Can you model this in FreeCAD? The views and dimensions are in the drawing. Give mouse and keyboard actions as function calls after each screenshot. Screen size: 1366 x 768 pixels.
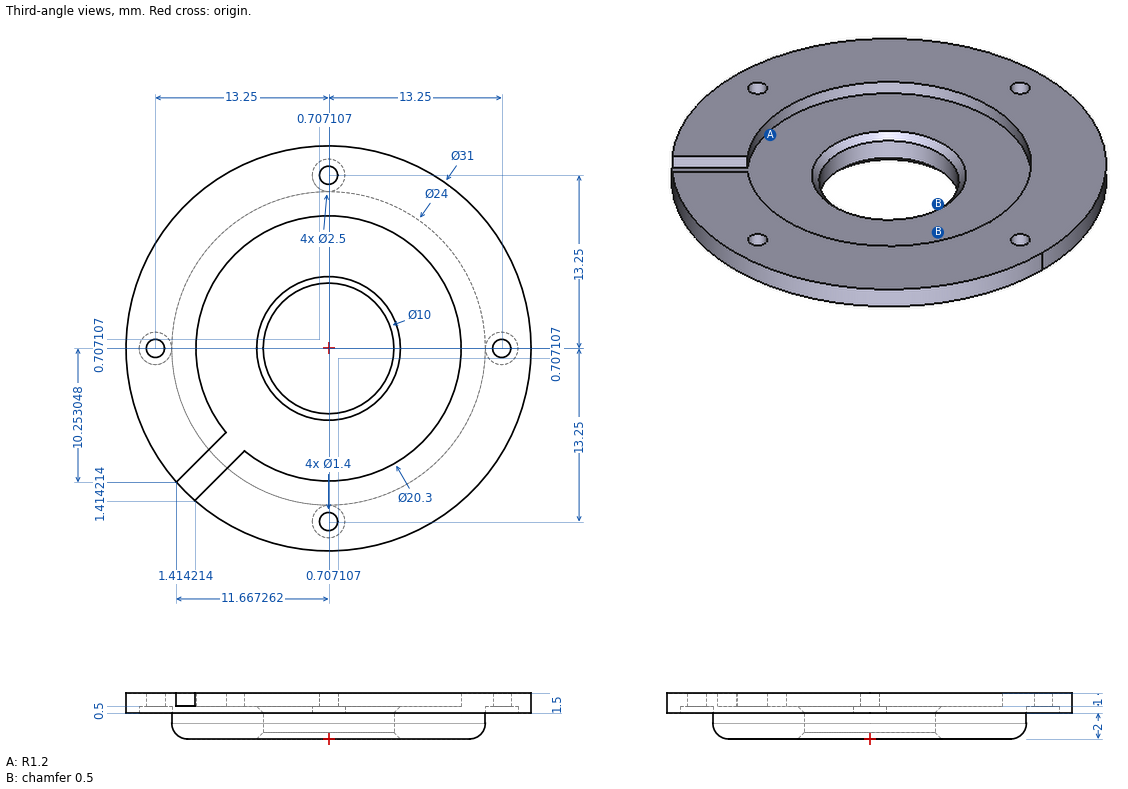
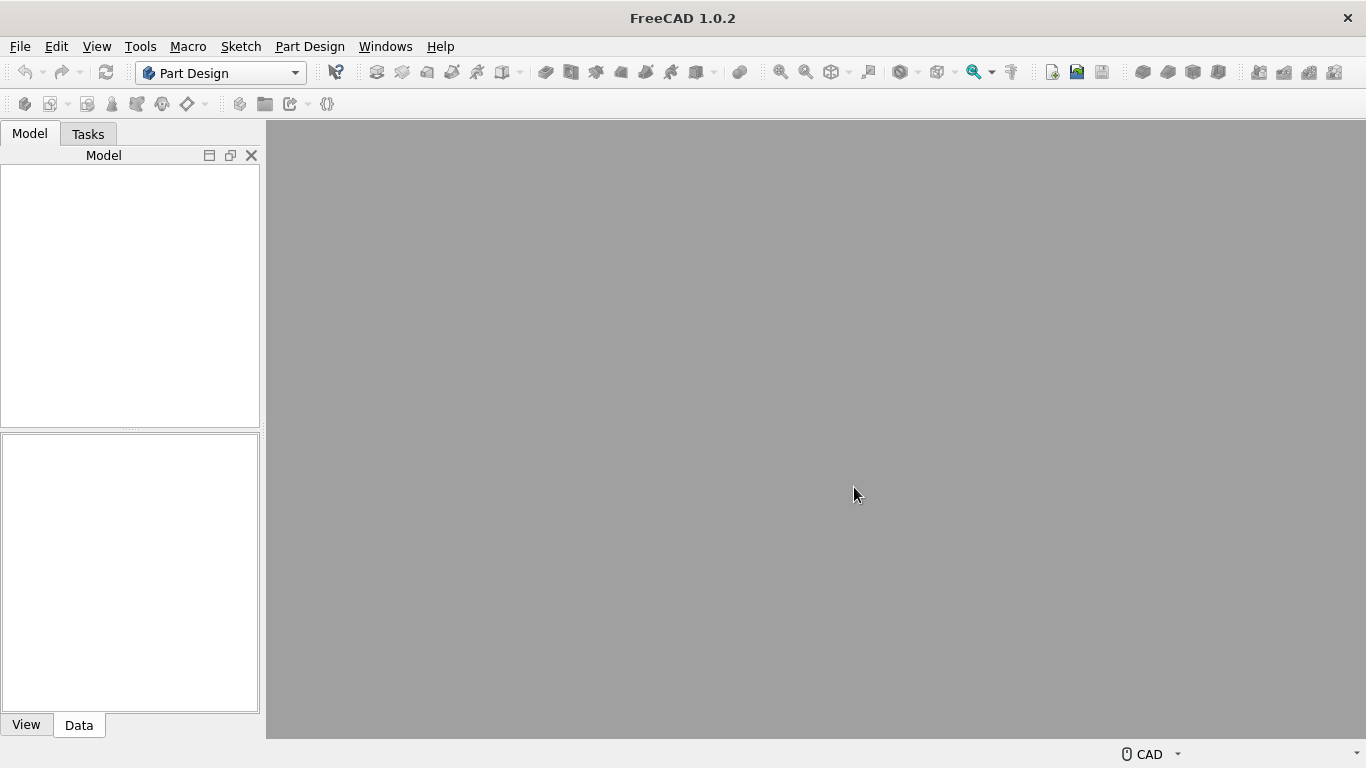
click(1052, 72)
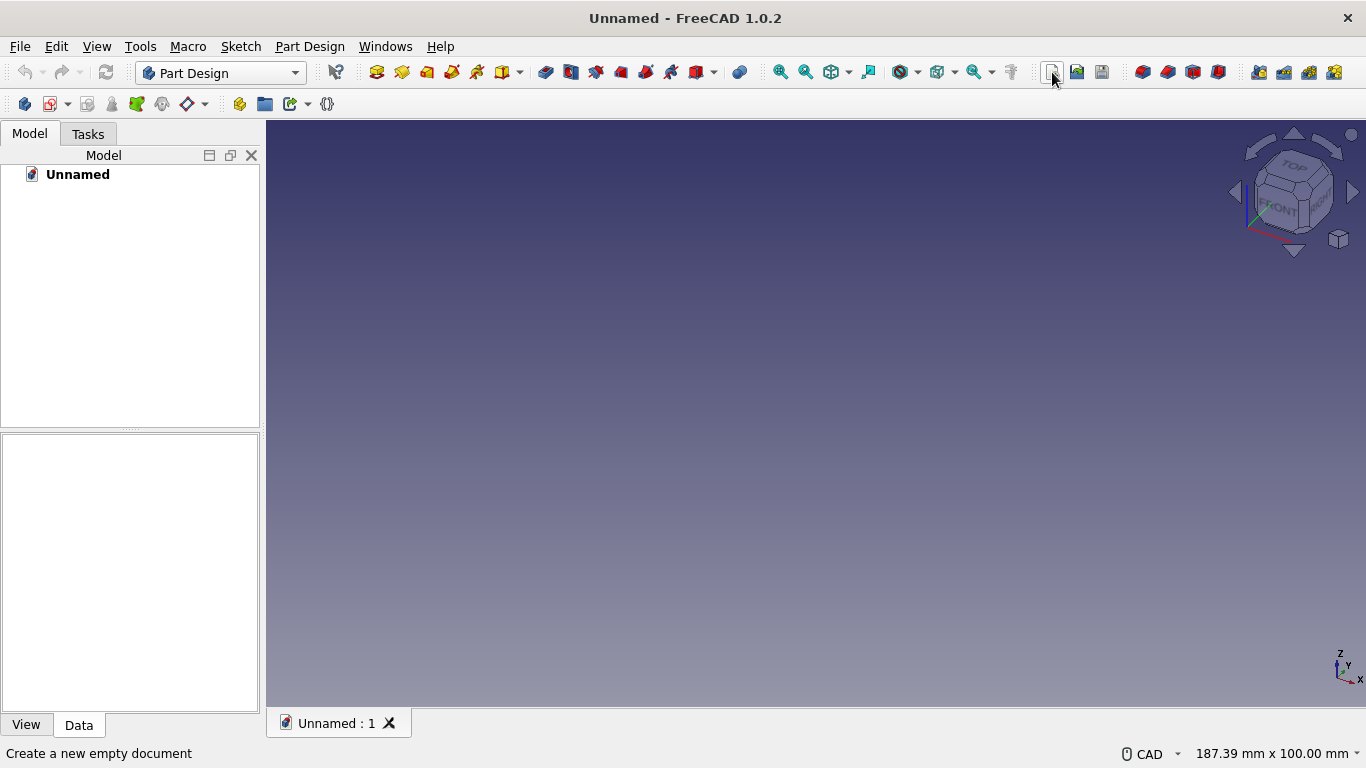
click(50, 104)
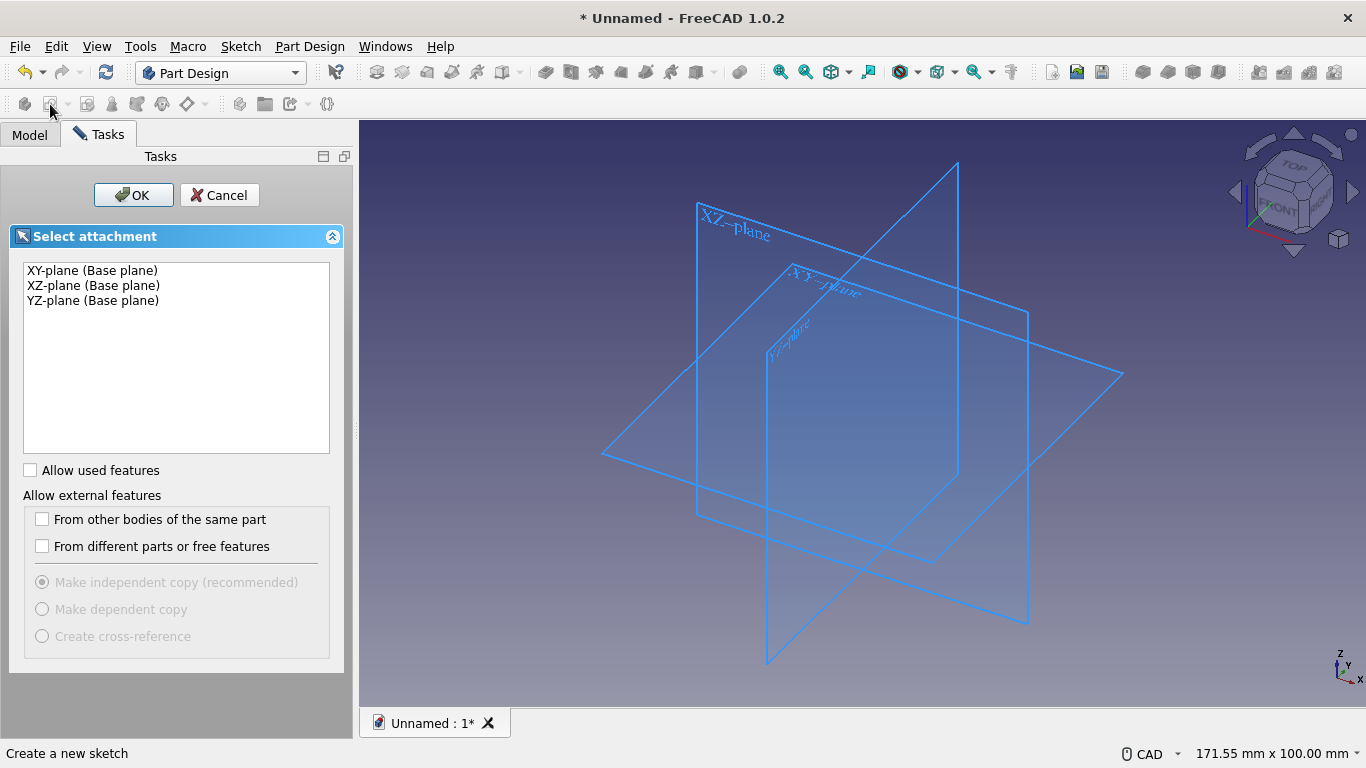
click(84, 270)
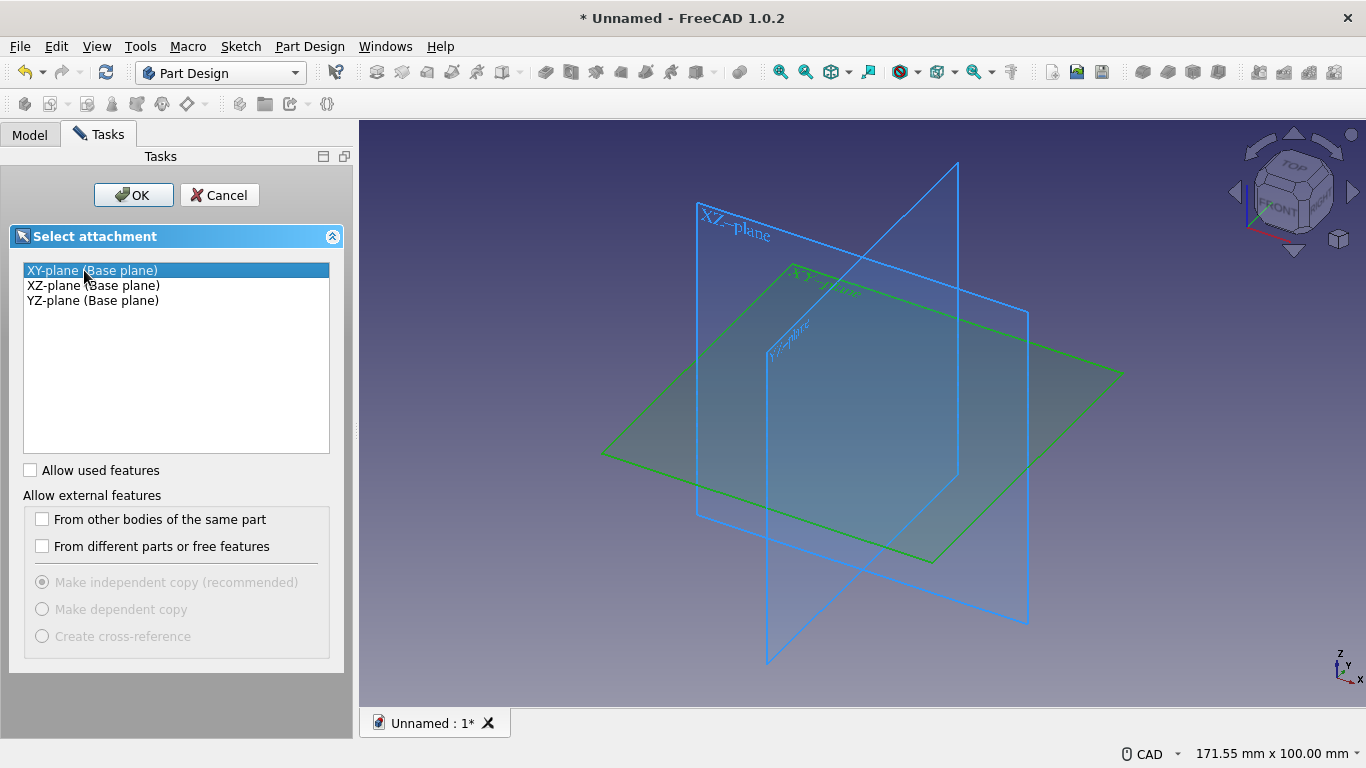
click(134, 195)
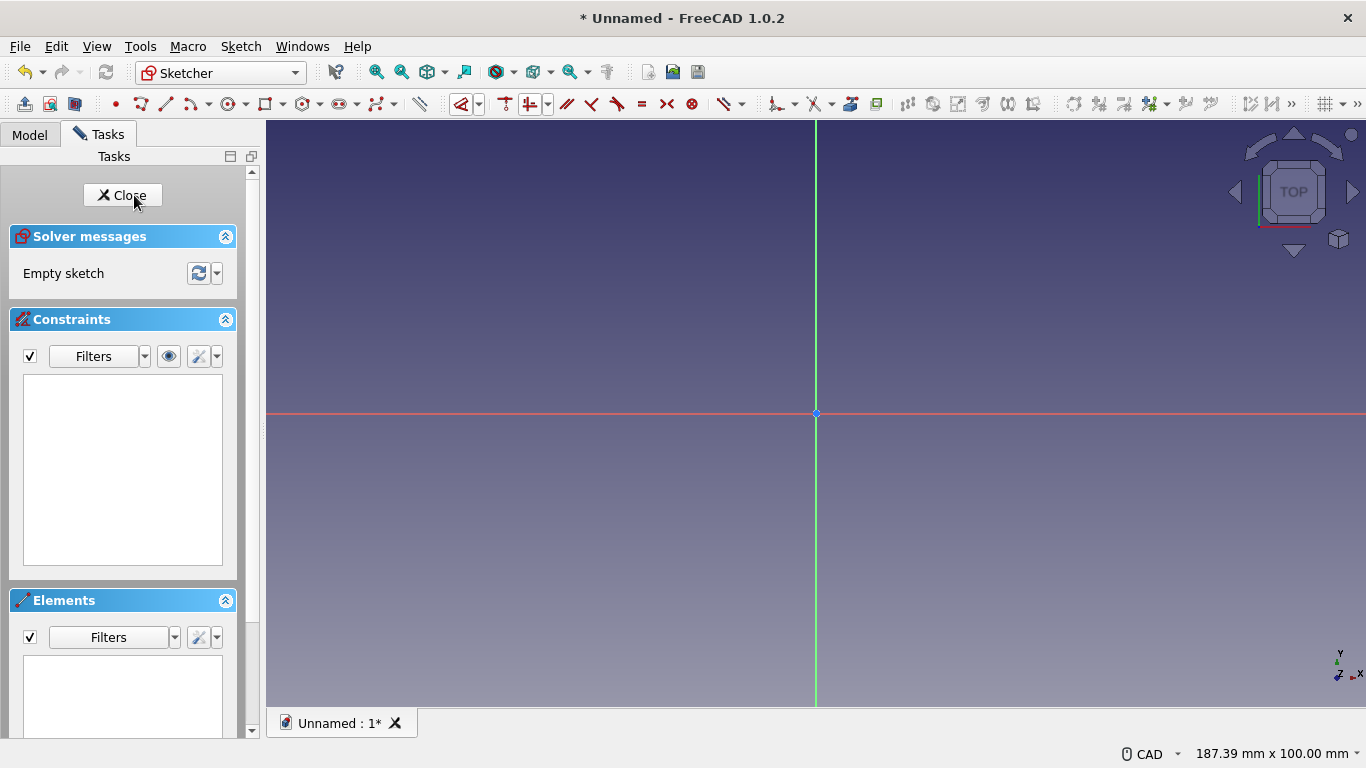
scroll(856, 414, up, 5)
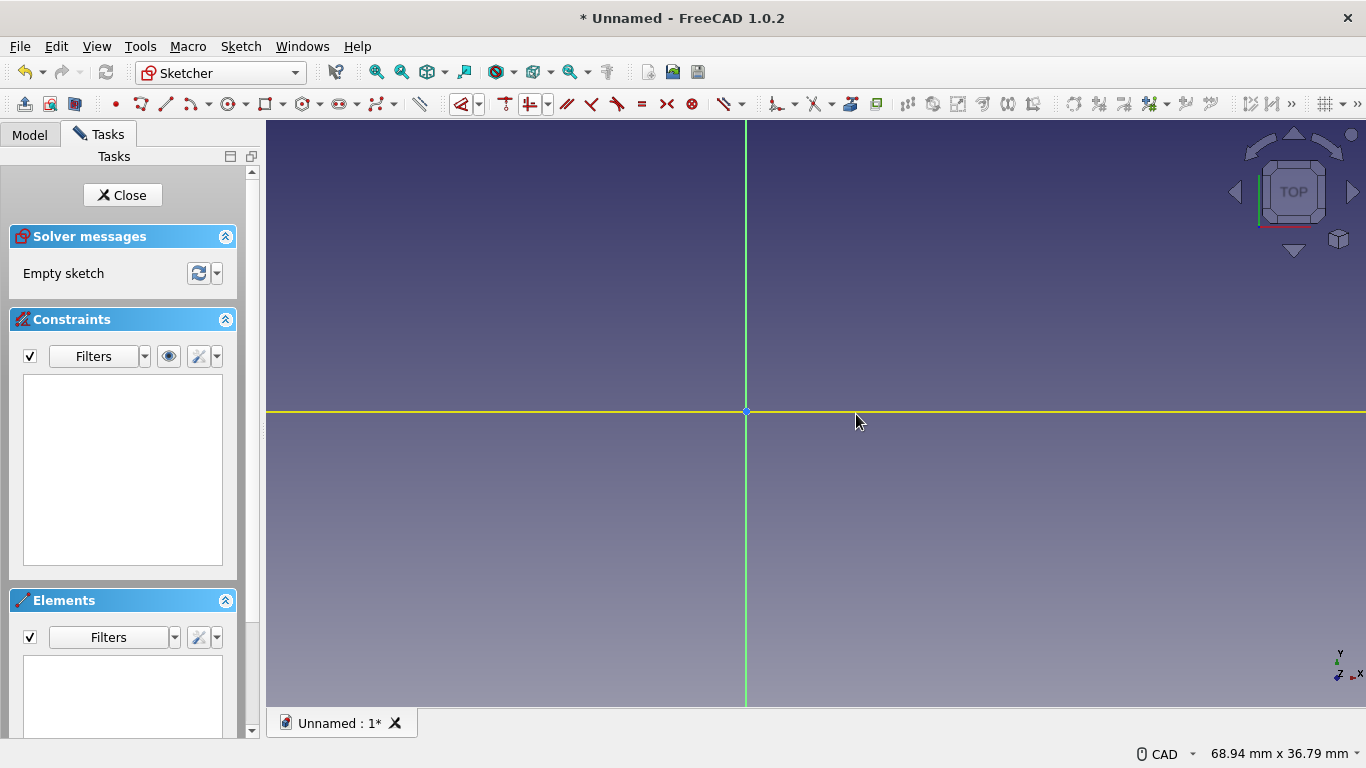
key(g)
key(c)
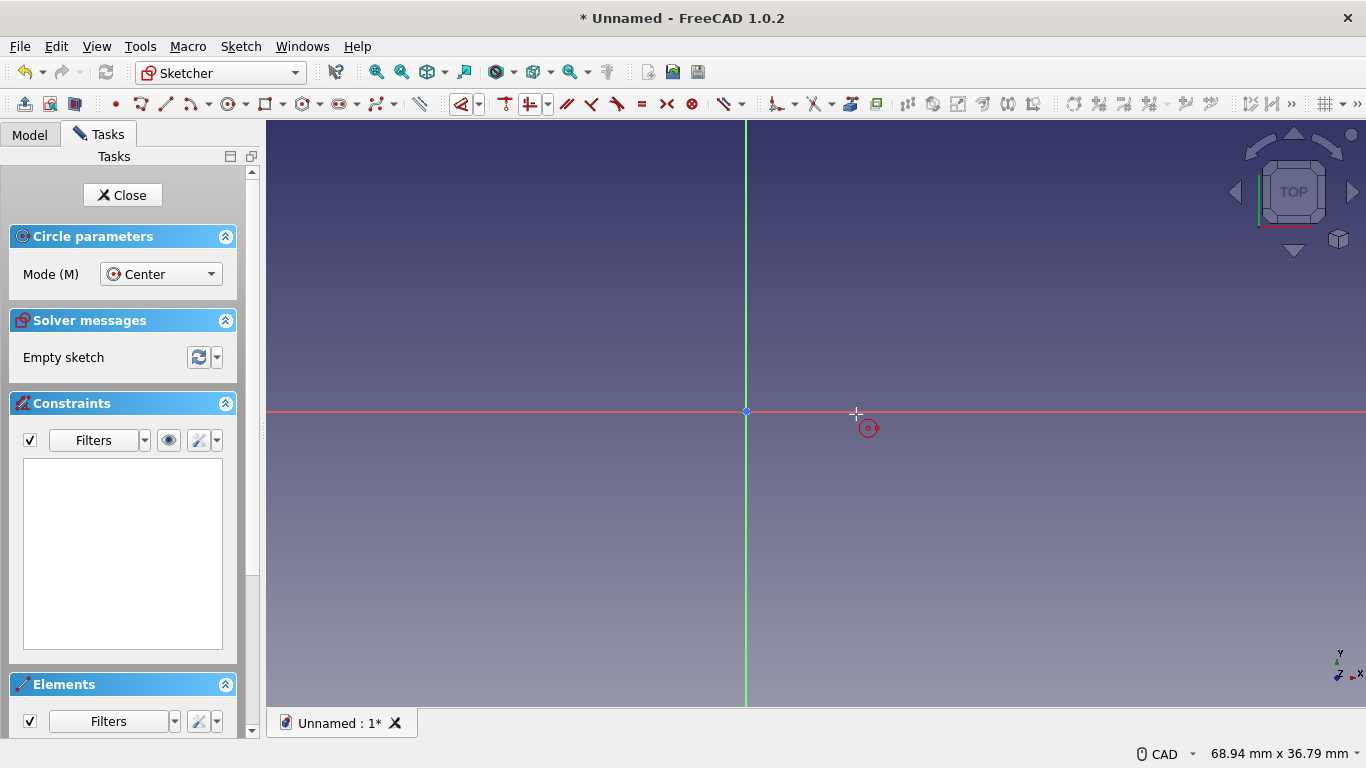
click(746, 412)
move(882, 276)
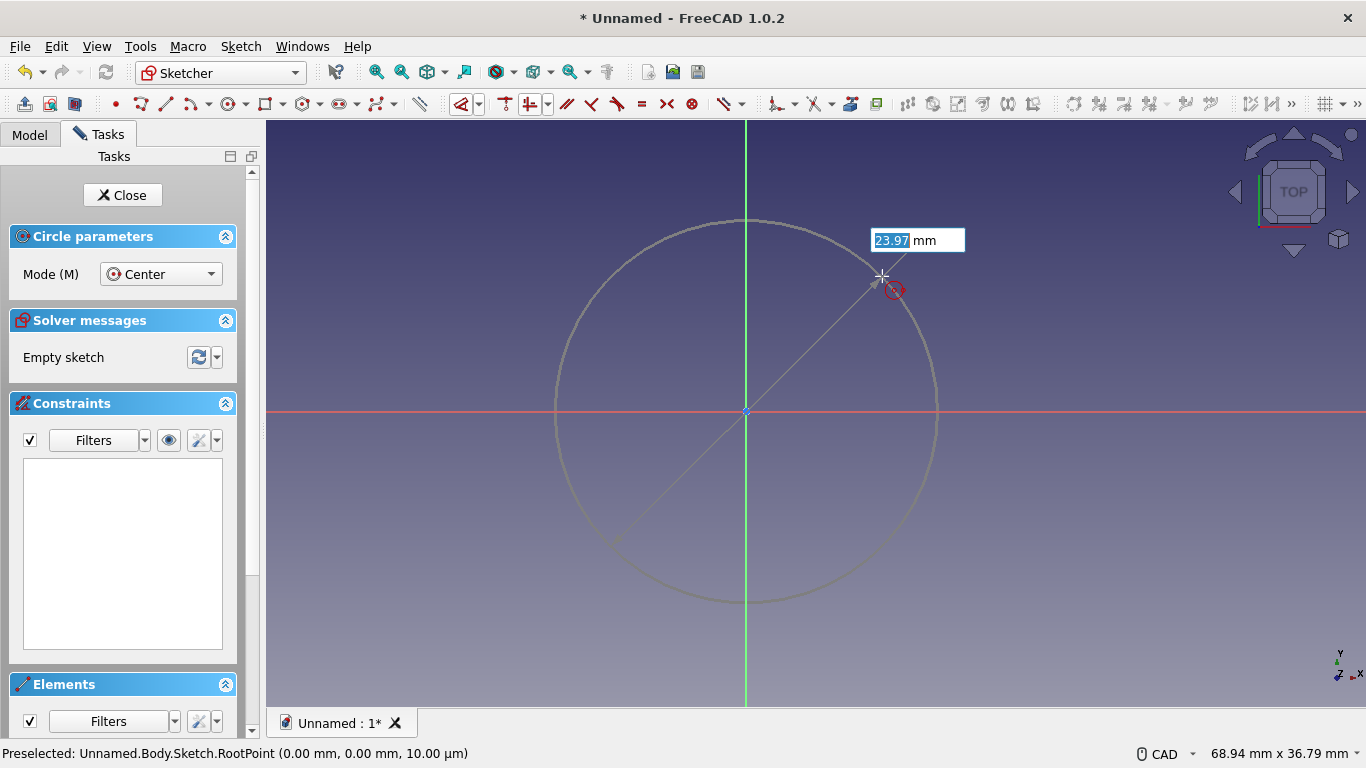
text(24)
key(Return)
key(Escape)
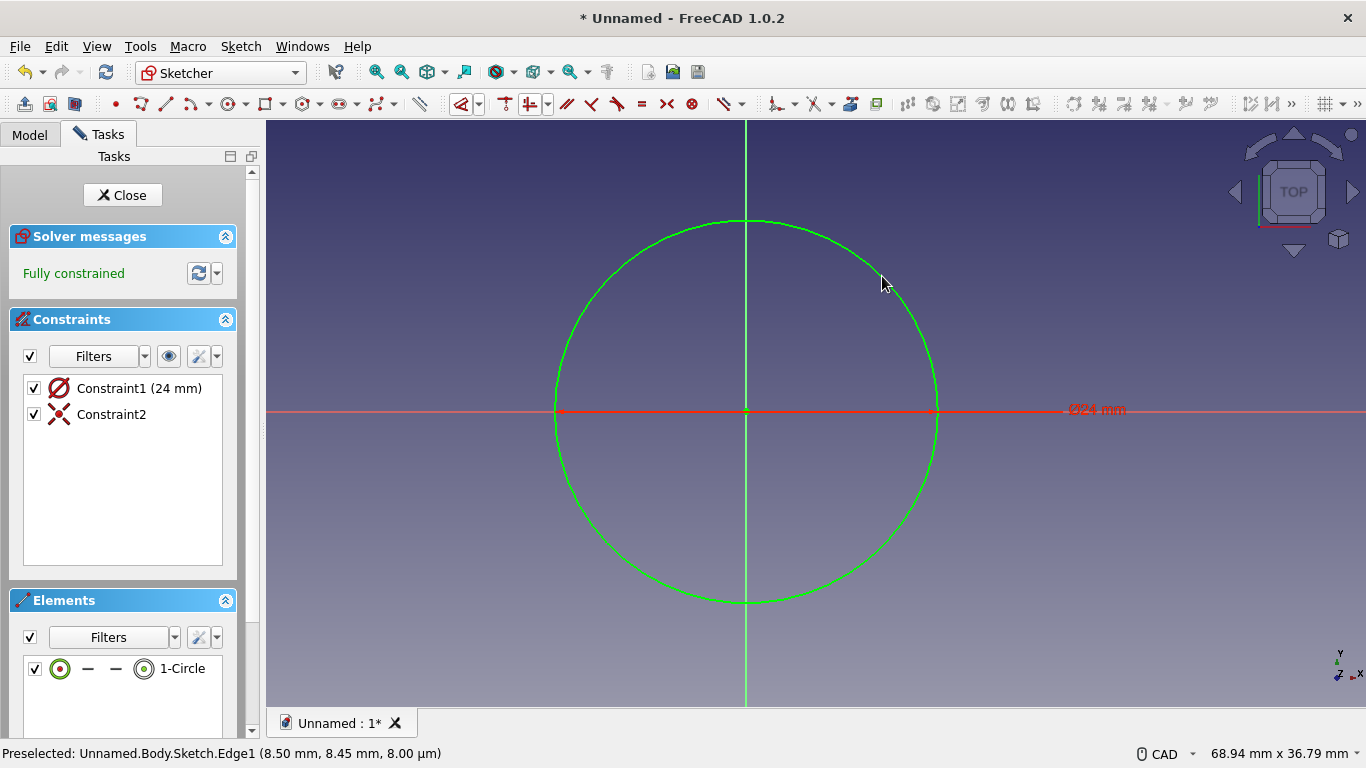
click(123, 195)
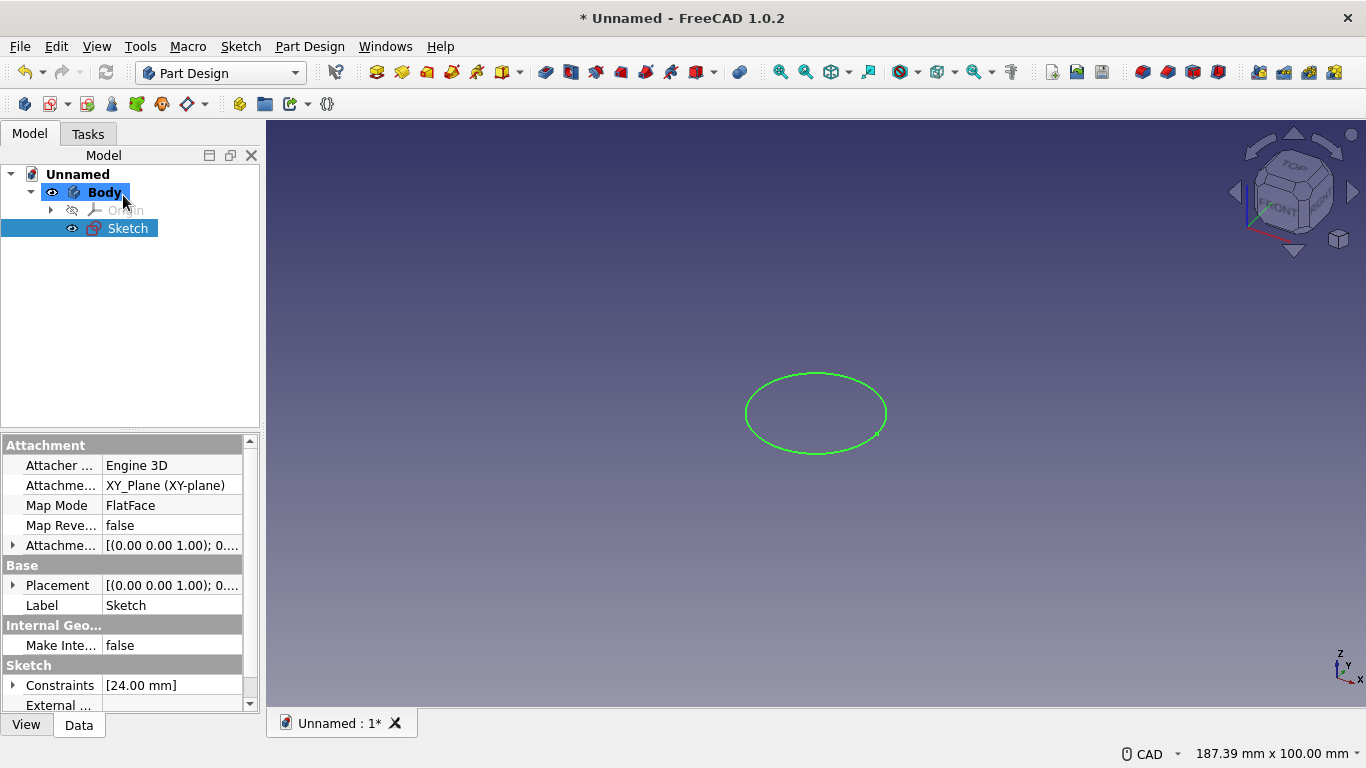
click(377, 72)